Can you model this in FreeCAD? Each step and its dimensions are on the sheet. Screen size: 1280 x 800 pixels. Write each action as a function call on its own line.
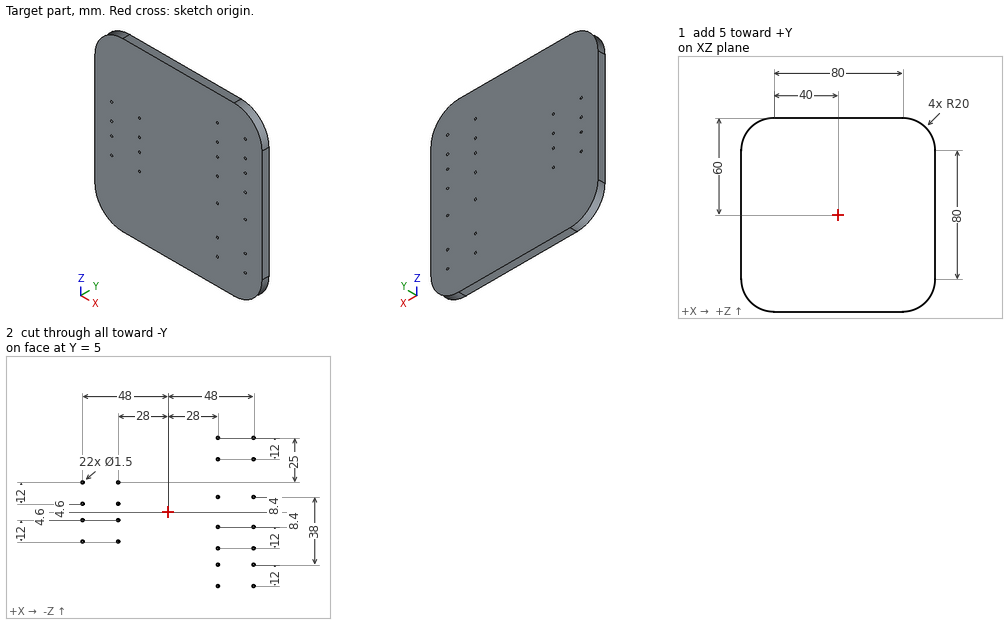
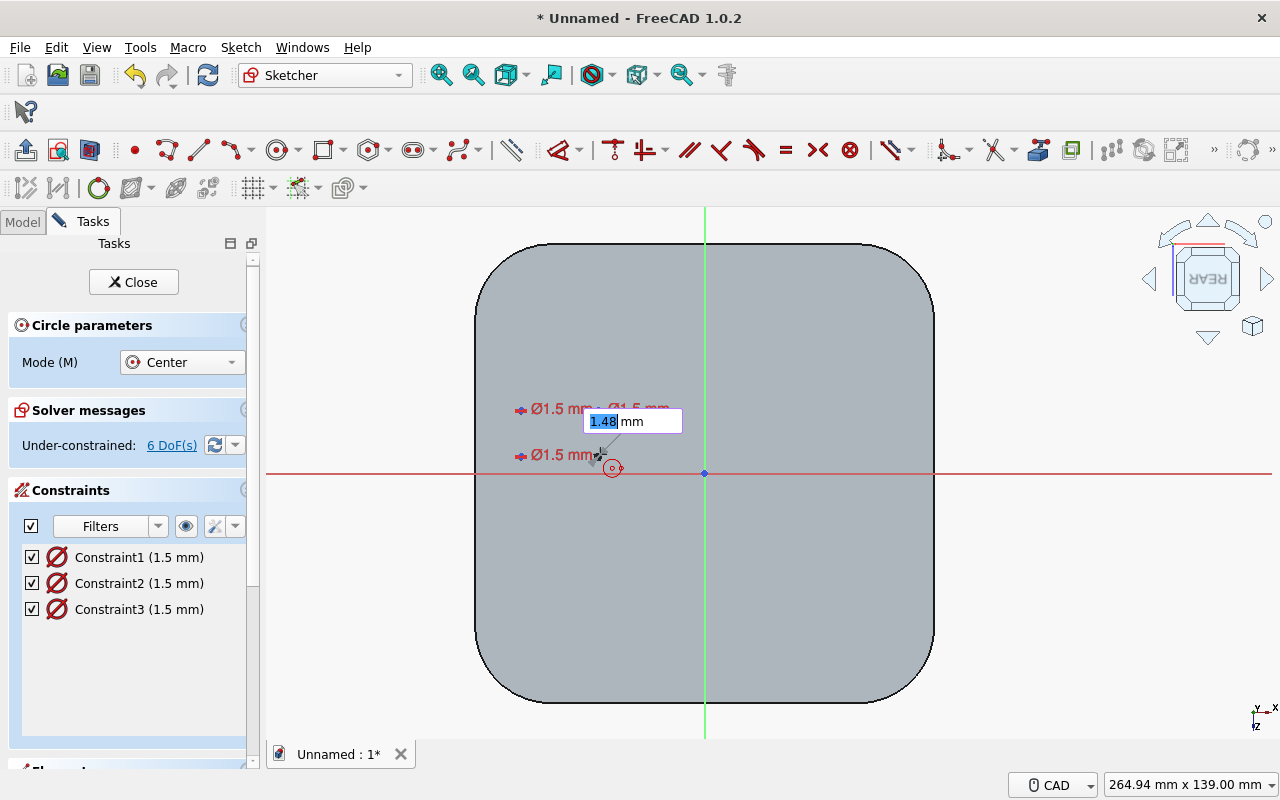
text(1.5)
key(Return)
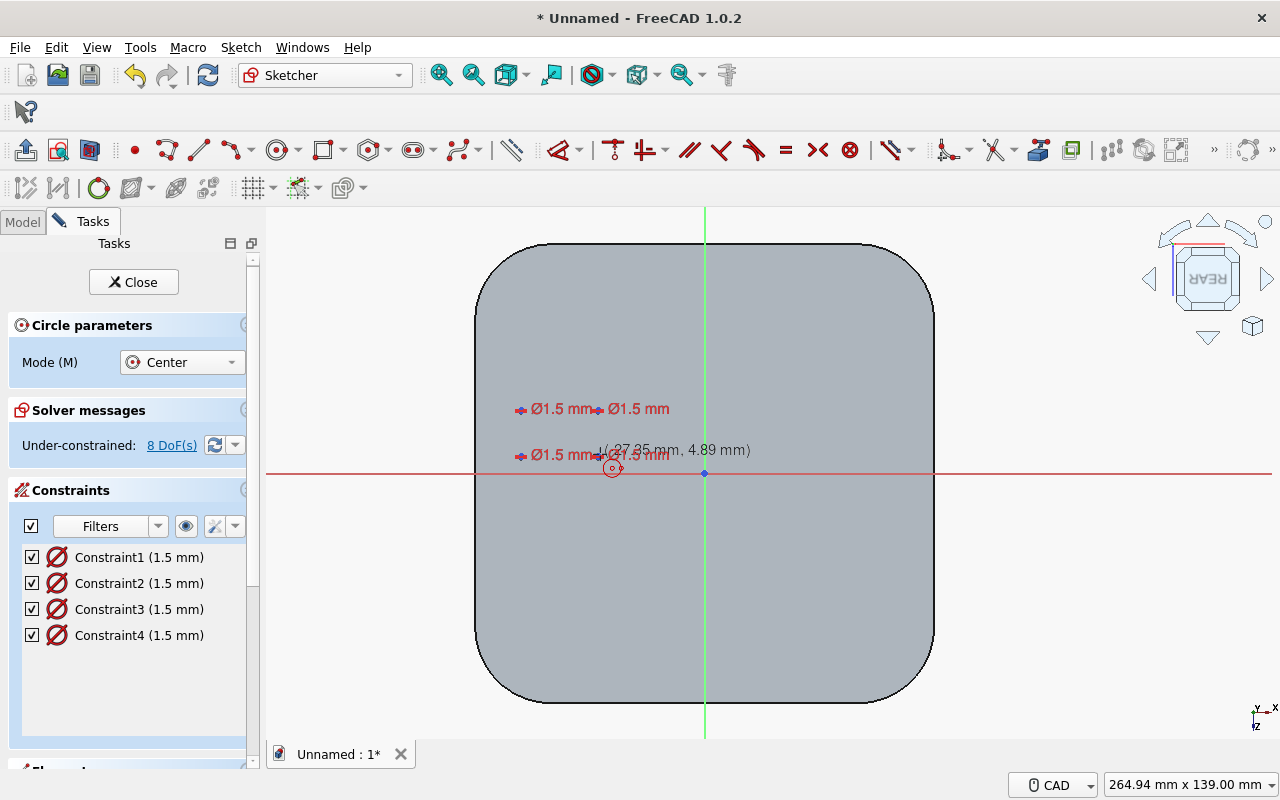
scroll(598, 491, up, 11)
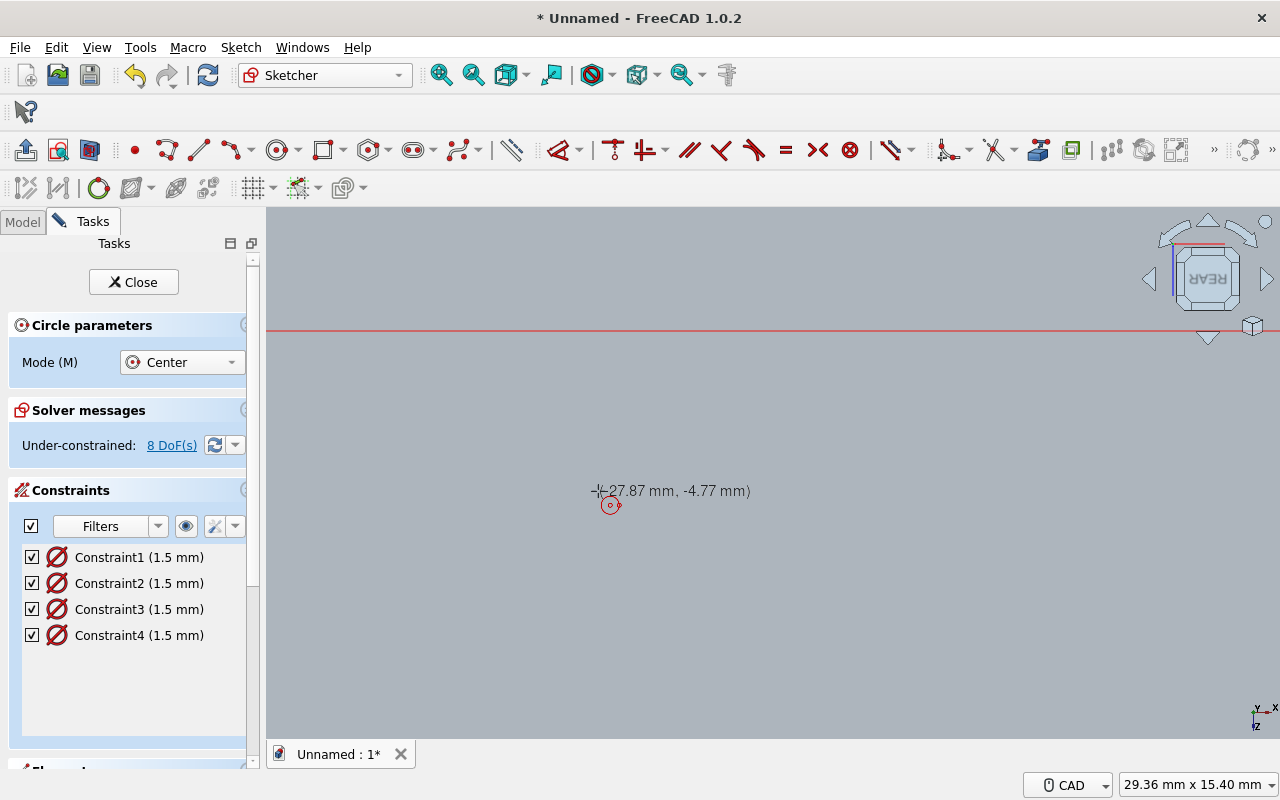
scroll(598, 491, down, 11)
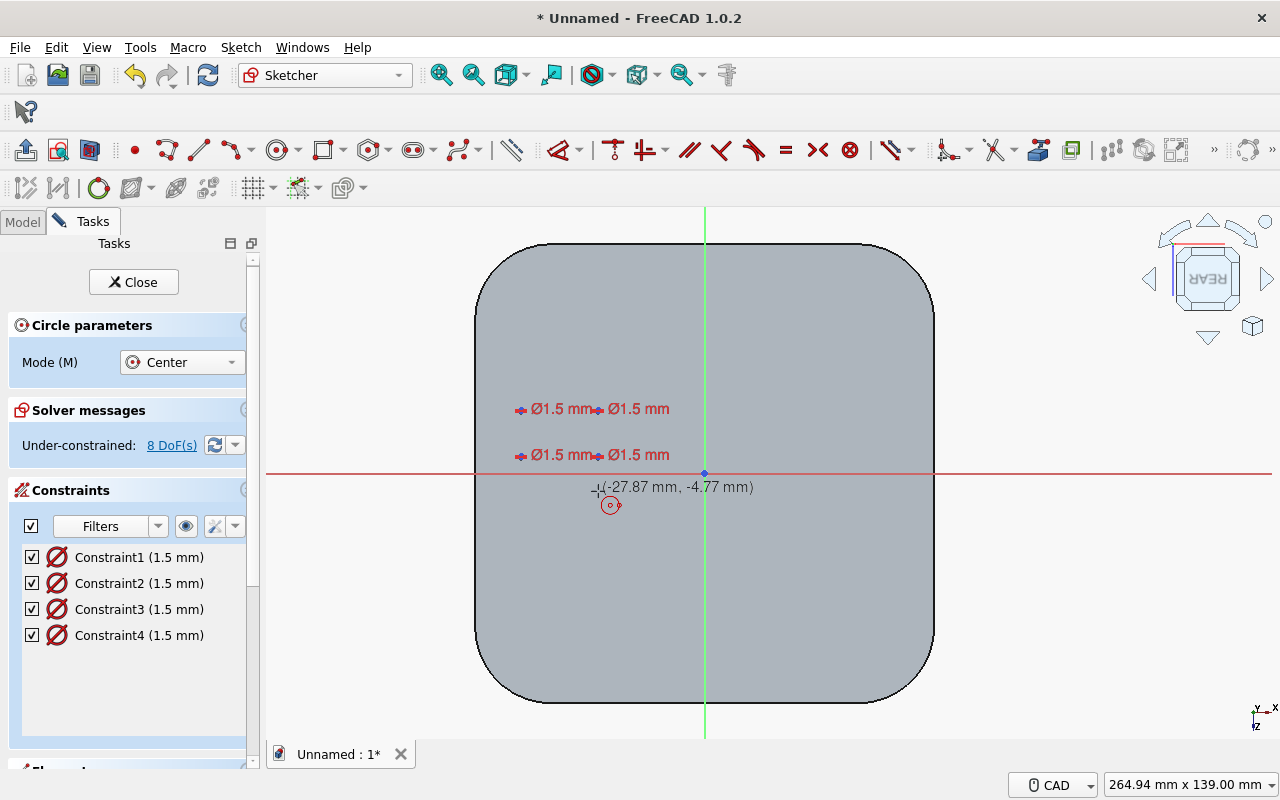
click(598, 491)
move(600, 489)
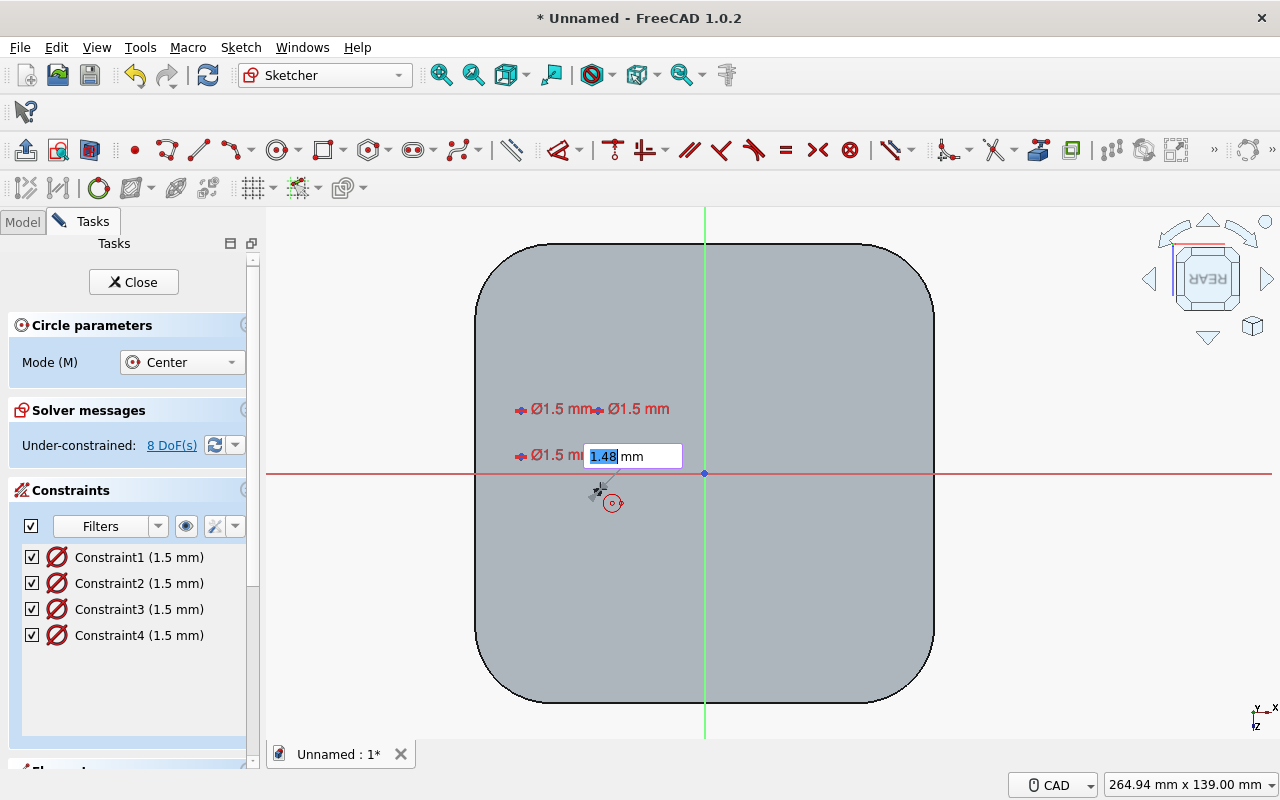
text(1.5)
key(Return)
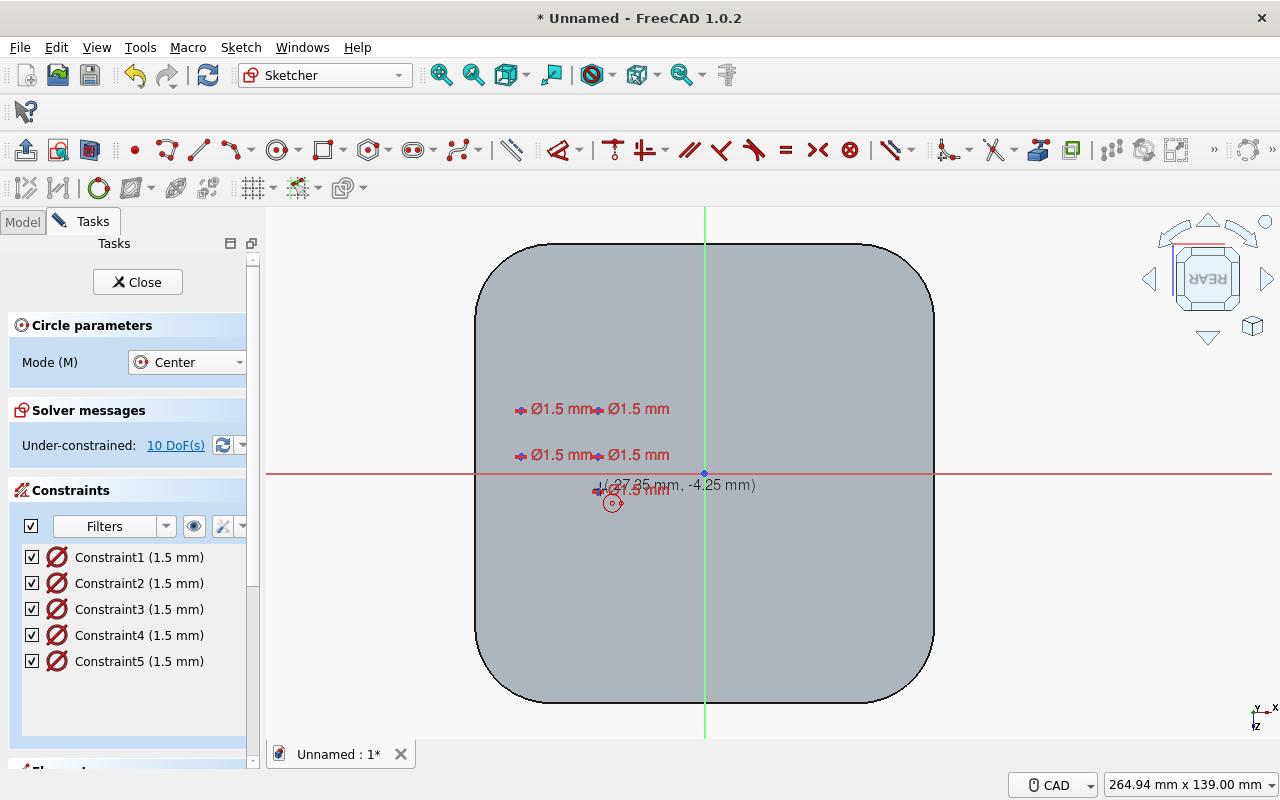
scroll(521, 491, up, 11)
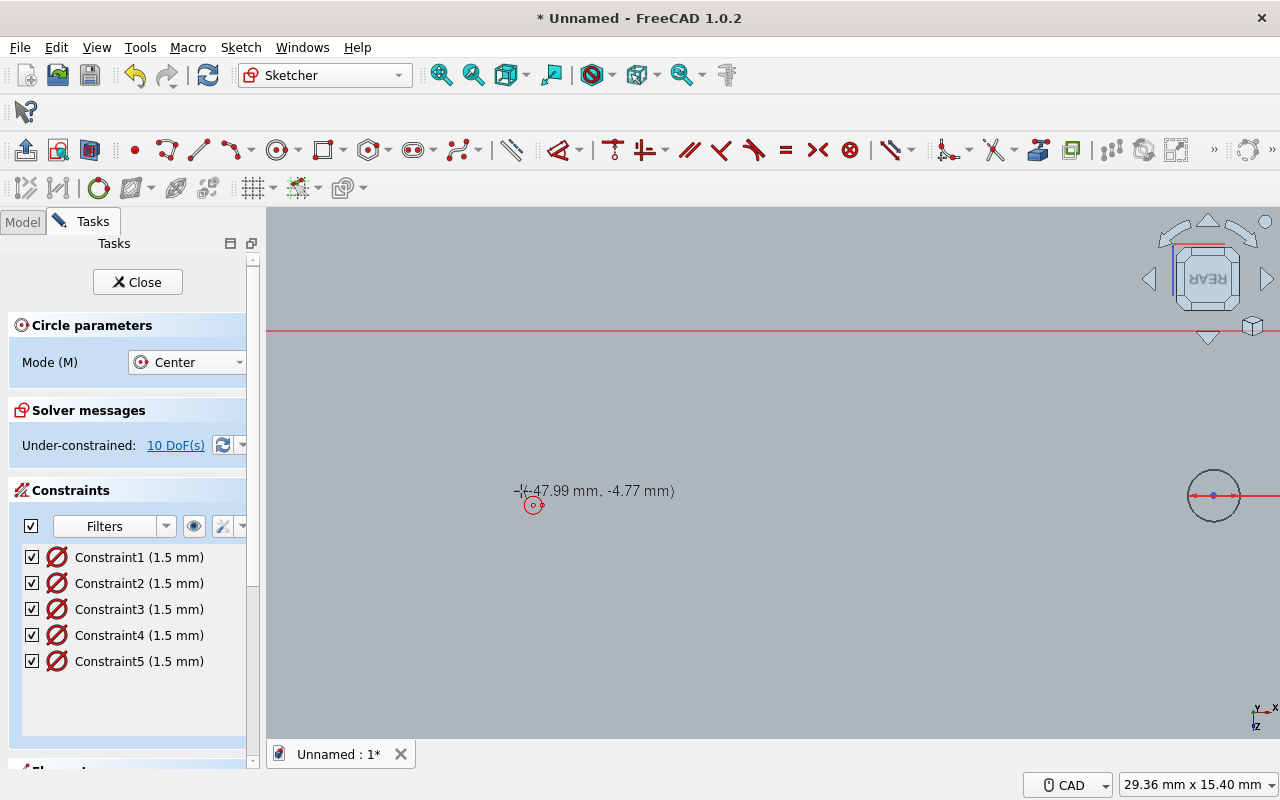
scroll(521, 491, down, 11)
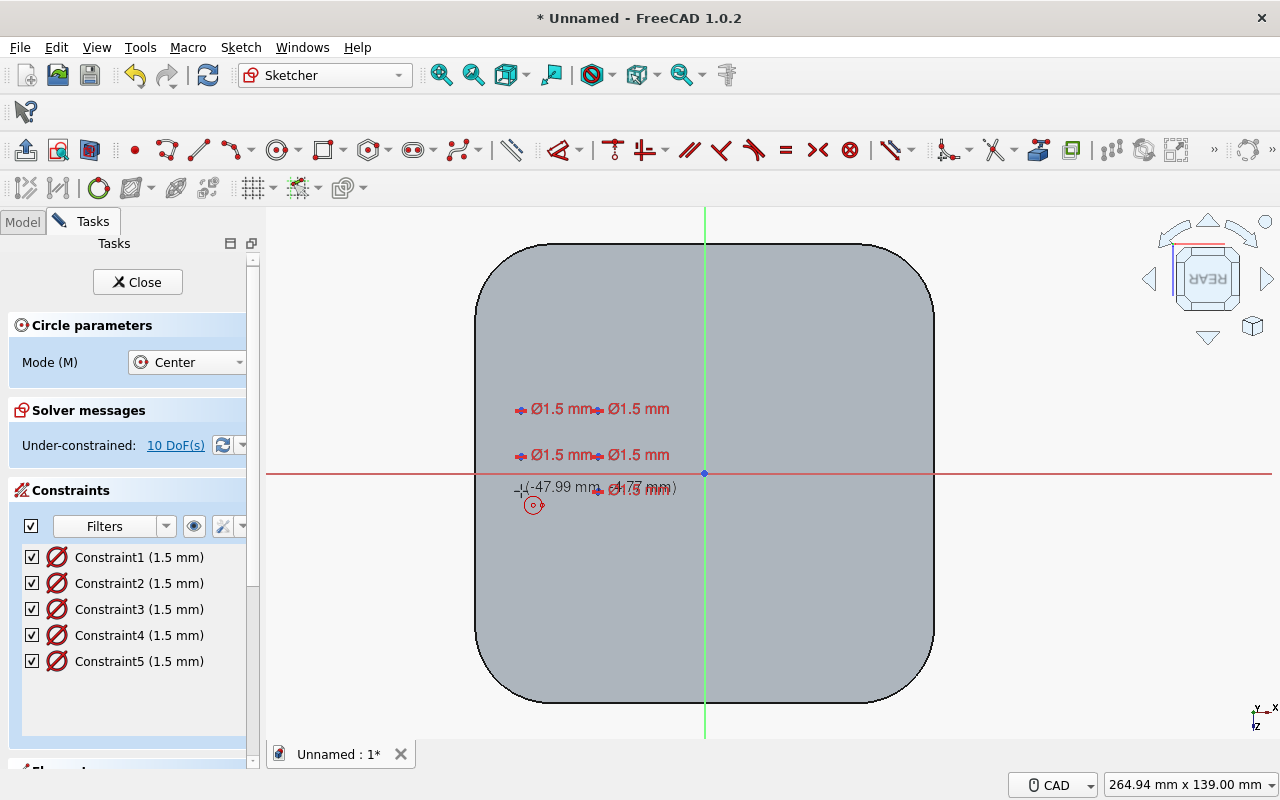
click(521, 491)
move(523, 489)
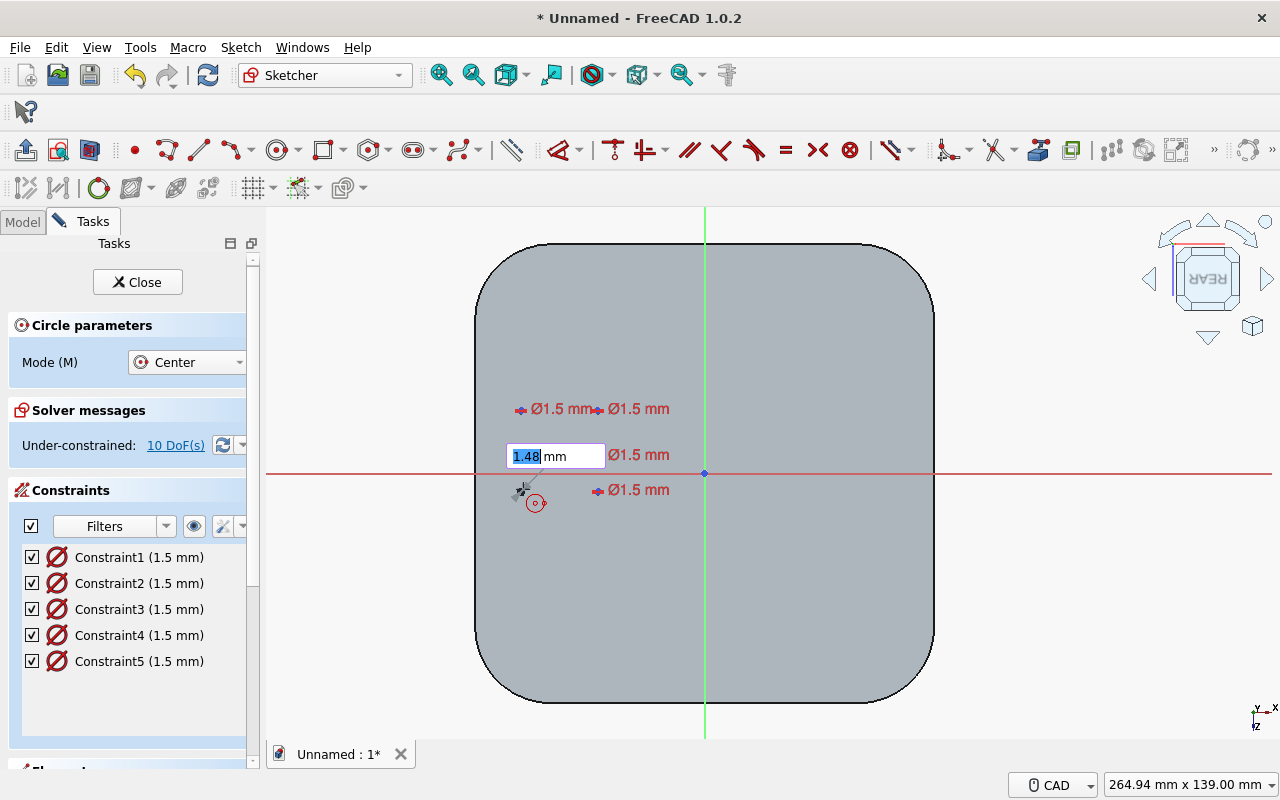
text(1.5)
key(Return)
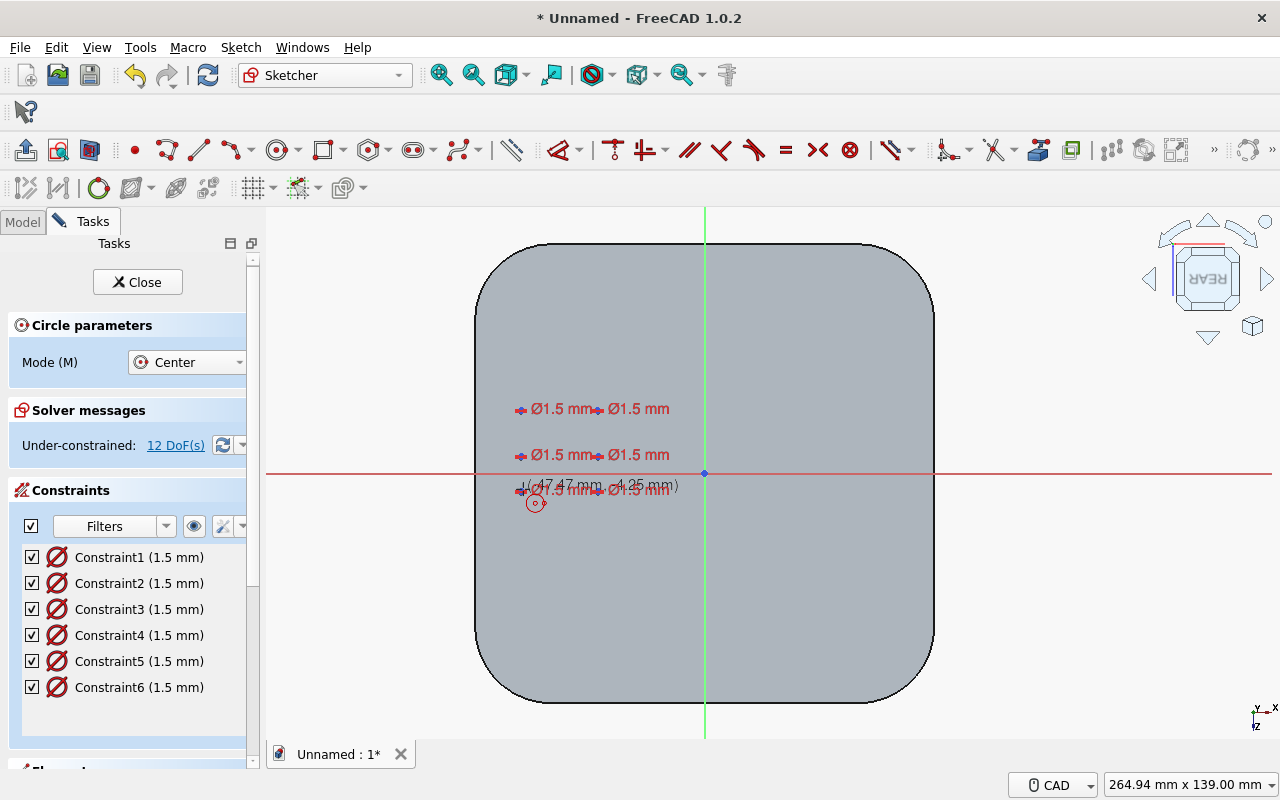
scroll(598, 537, up, 11)